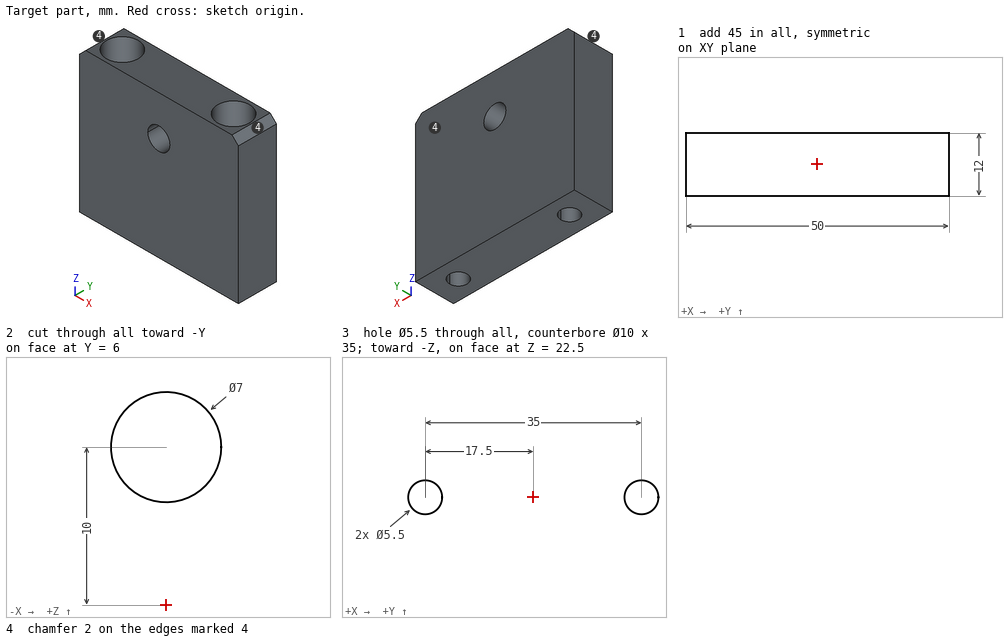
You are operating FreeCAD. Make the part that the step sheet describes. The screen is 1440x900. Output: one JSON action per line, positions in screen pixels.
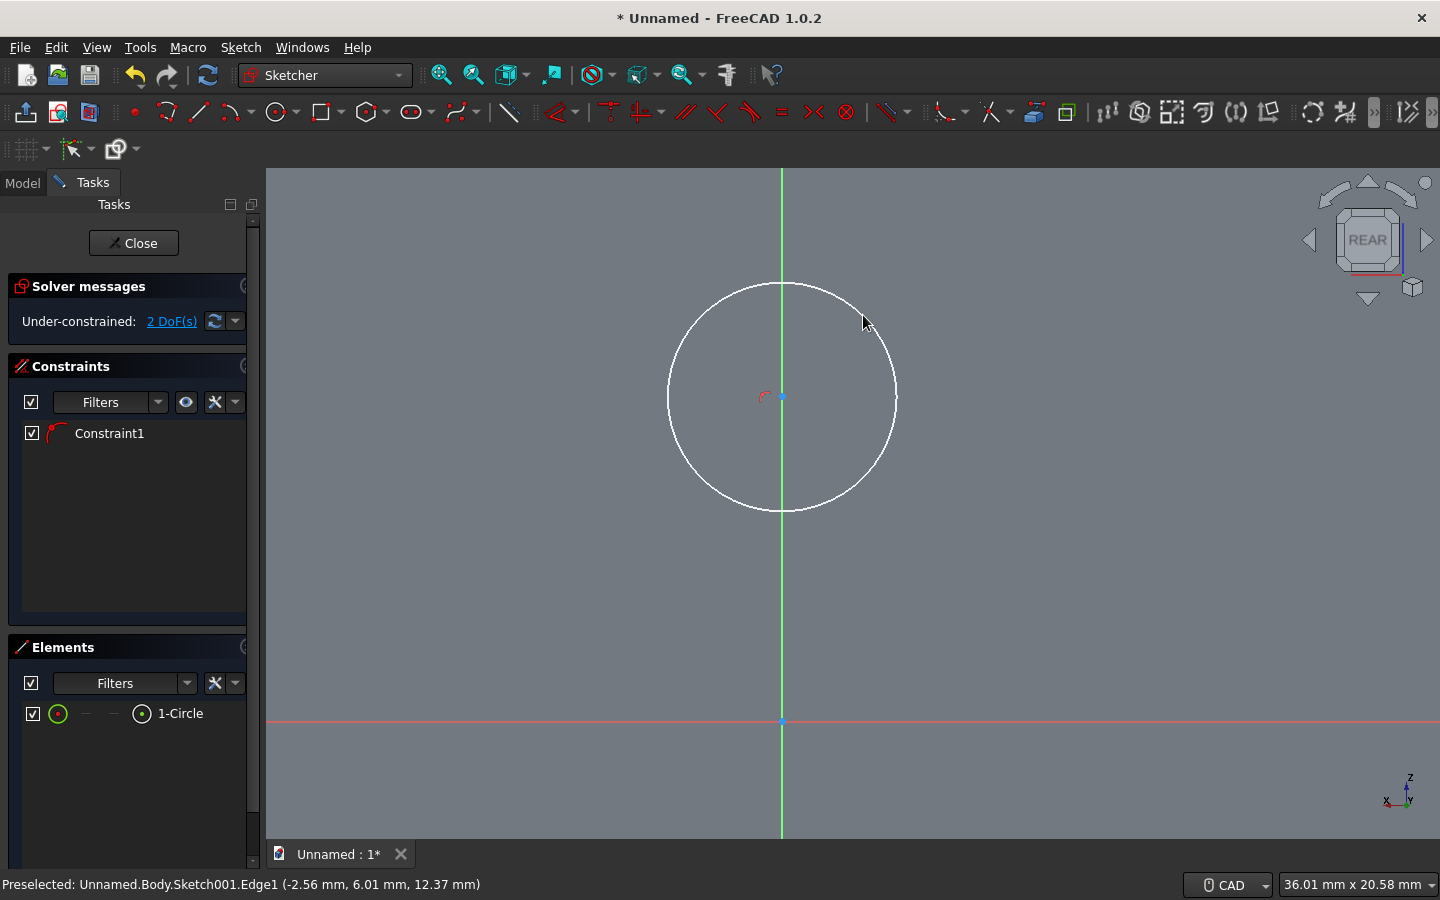
{"action": "left_click", "coordinate": [556, 112]}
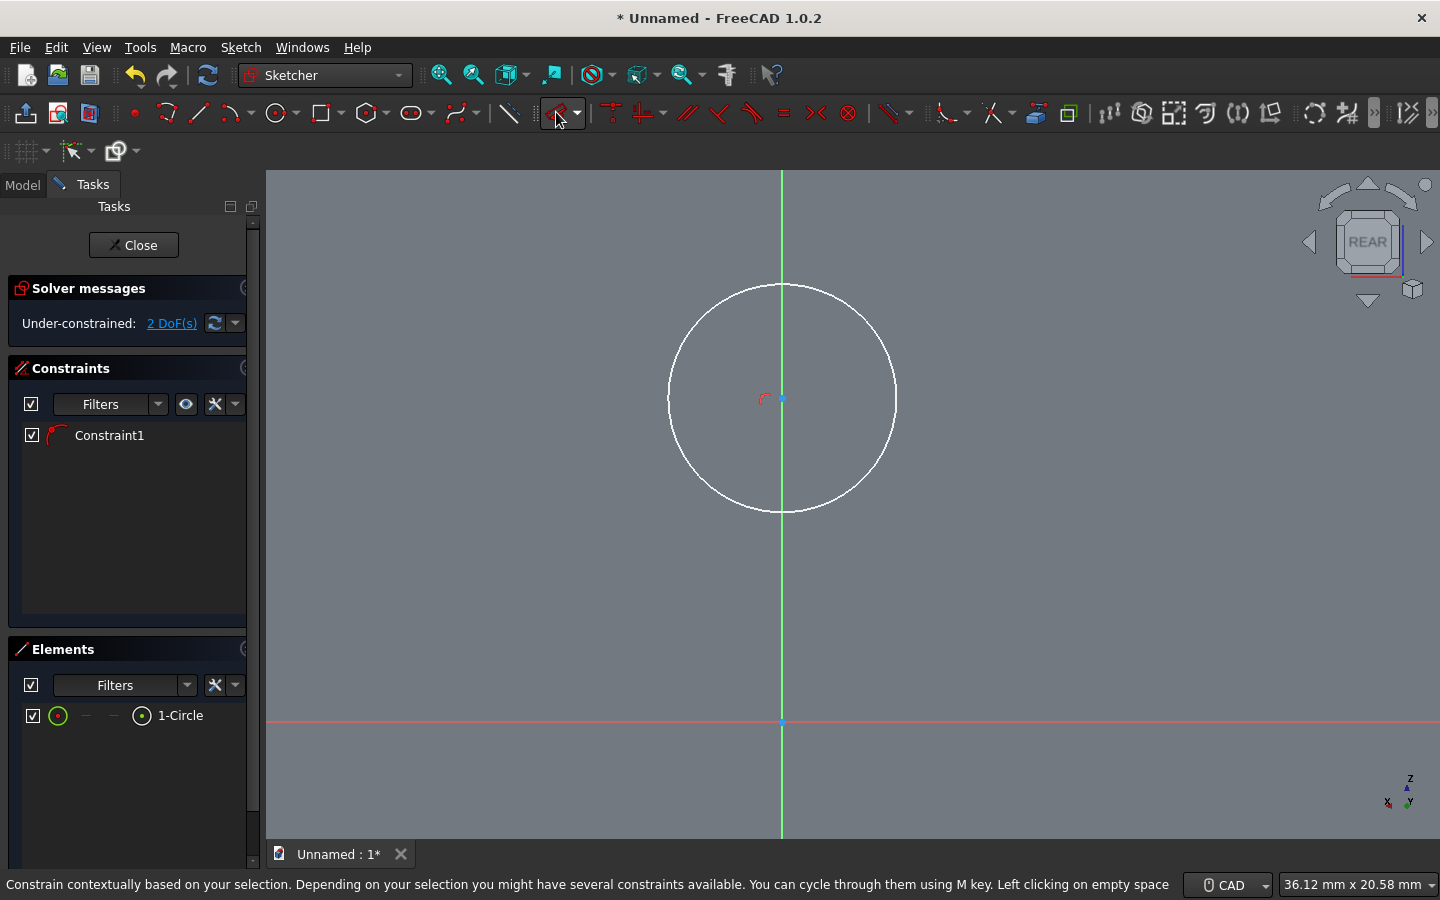
{"action": "left_click", "coordinate": [863, 317]}
{"action": "left_click", "coordinate": [886, 294]}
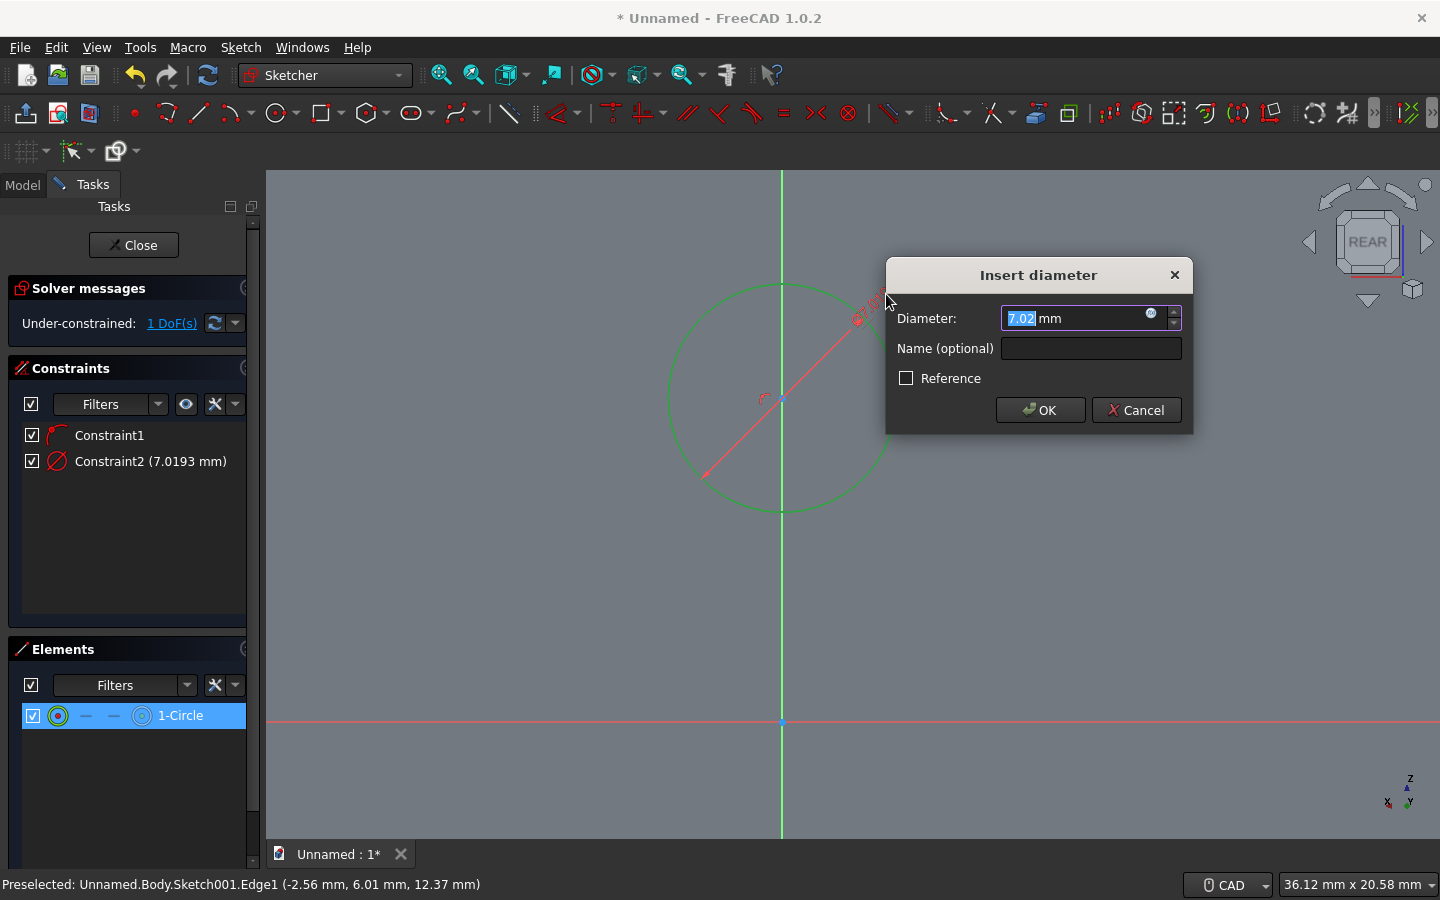
{"action": "type", "text": "7"}
{"action": "key", "text": "Return"}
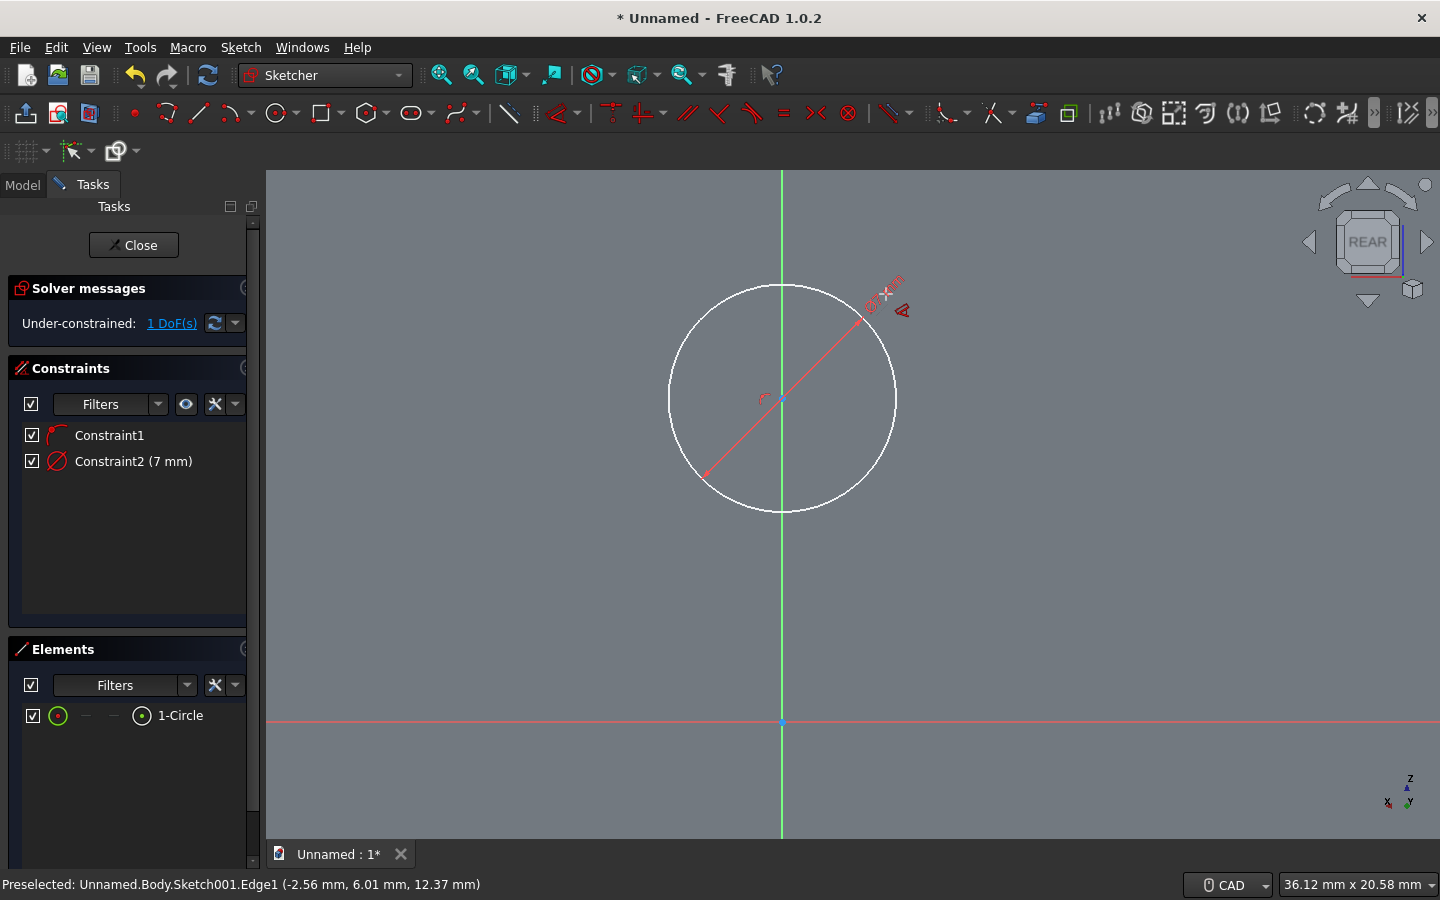
{"action": "left_click", "coordinate": [782, 398]}
{"action": "left_click", "coordinate": [816, 560]}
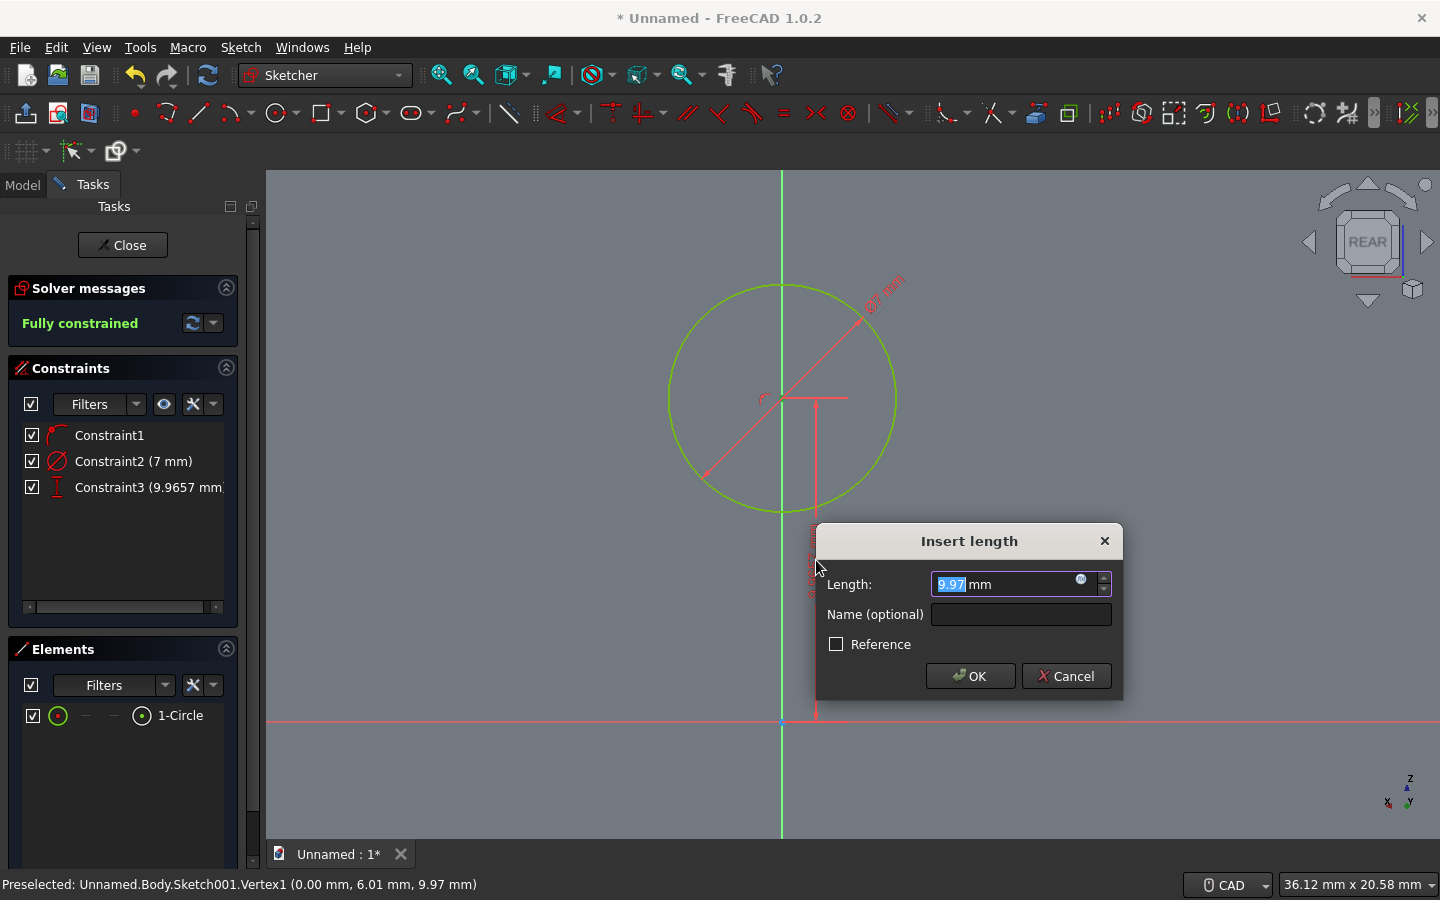
{"action": "type", "text": "10"}
{"action": "key", "text": "Return"}
{"action": "key", "text": "Escape"}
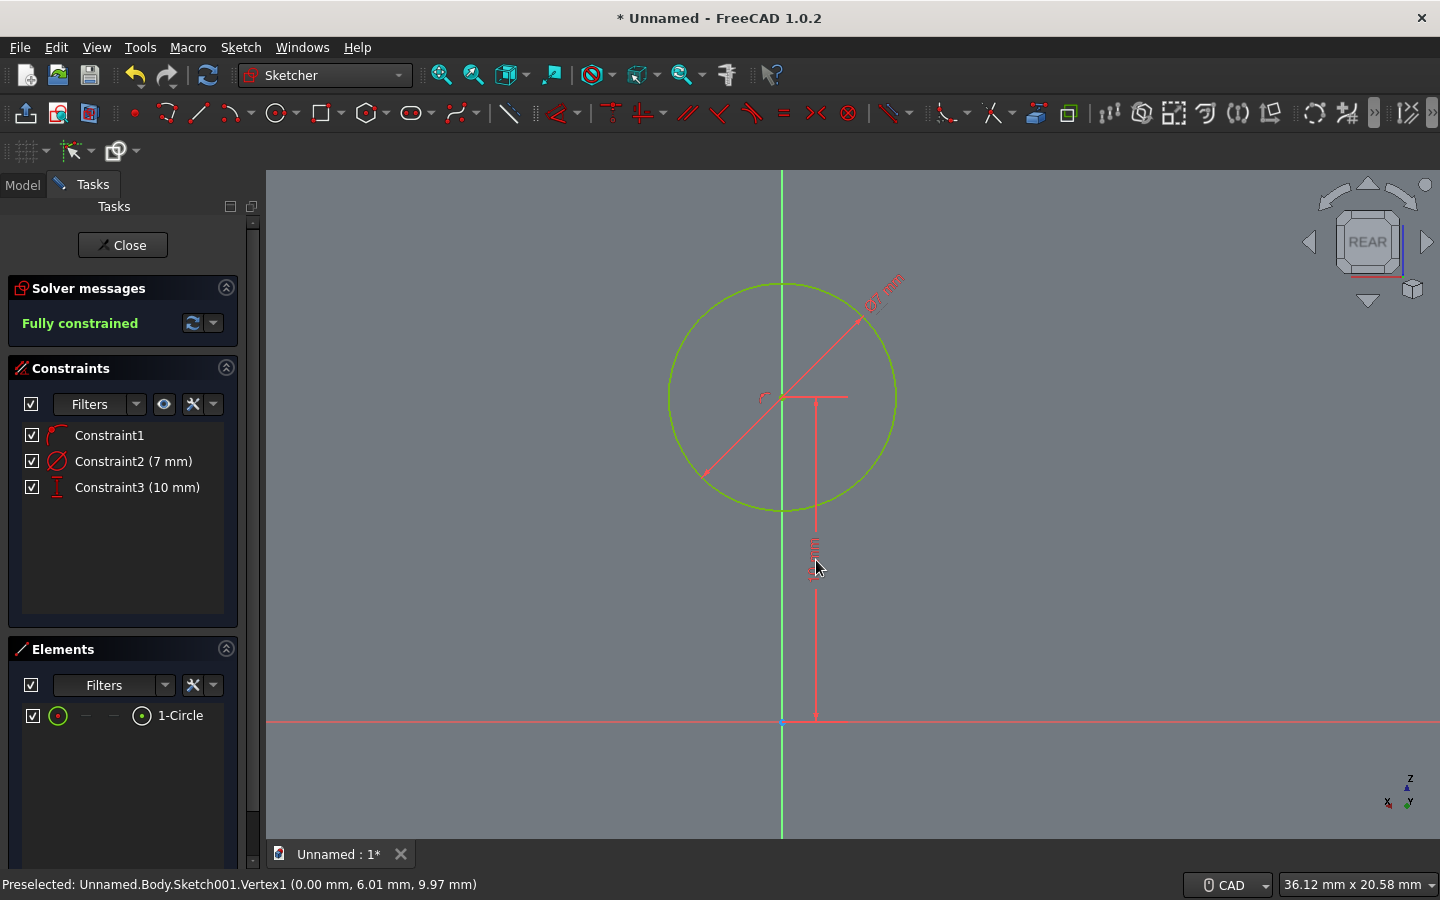
{"action": "left_click", "coordinate": [123, 245]}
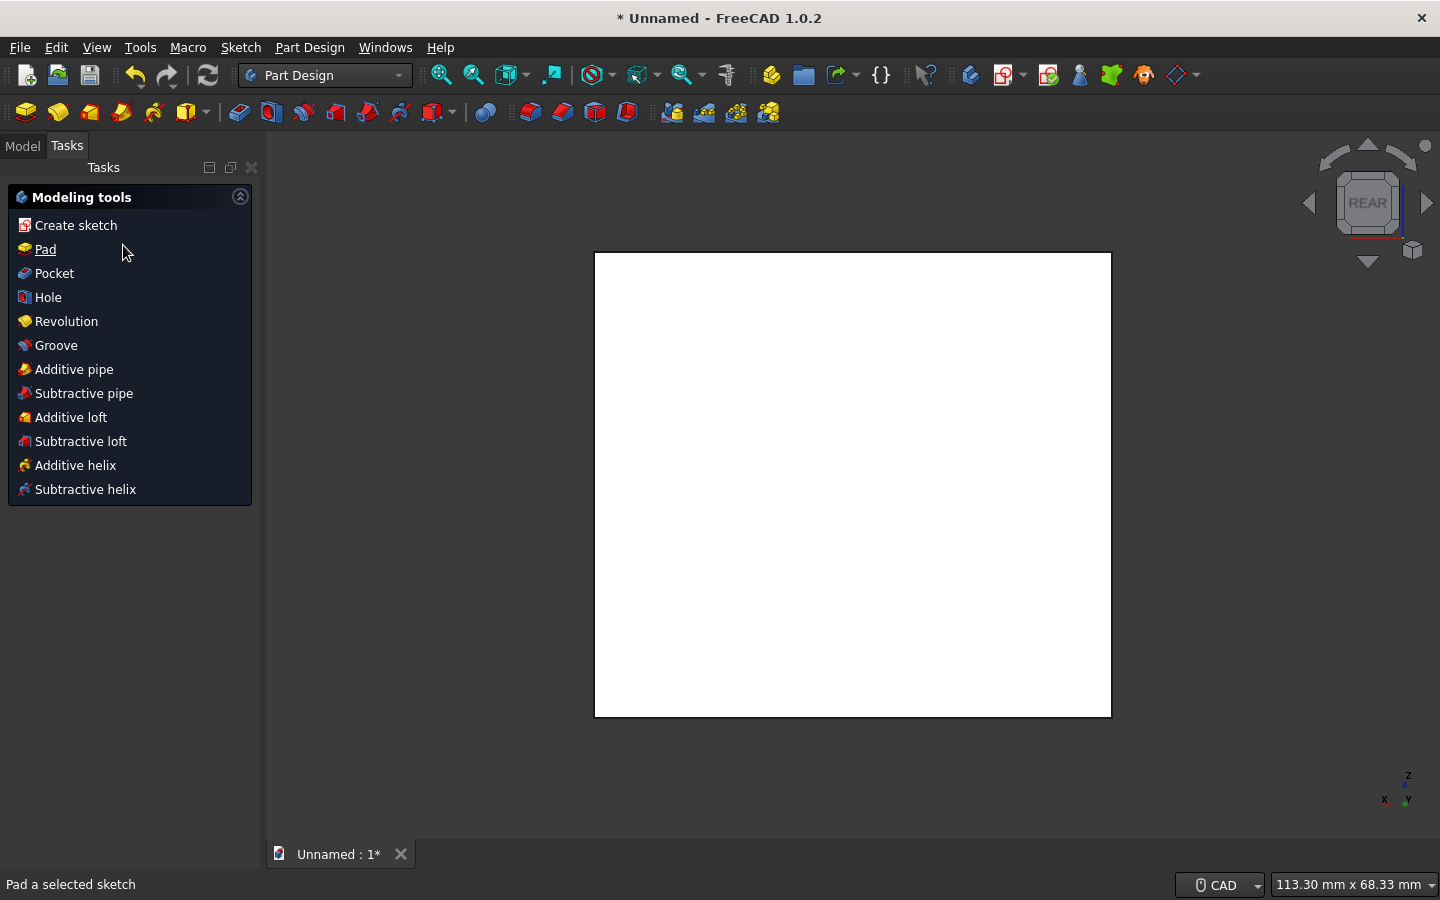
{"action": "left_click", "coordinate": [240, 112]}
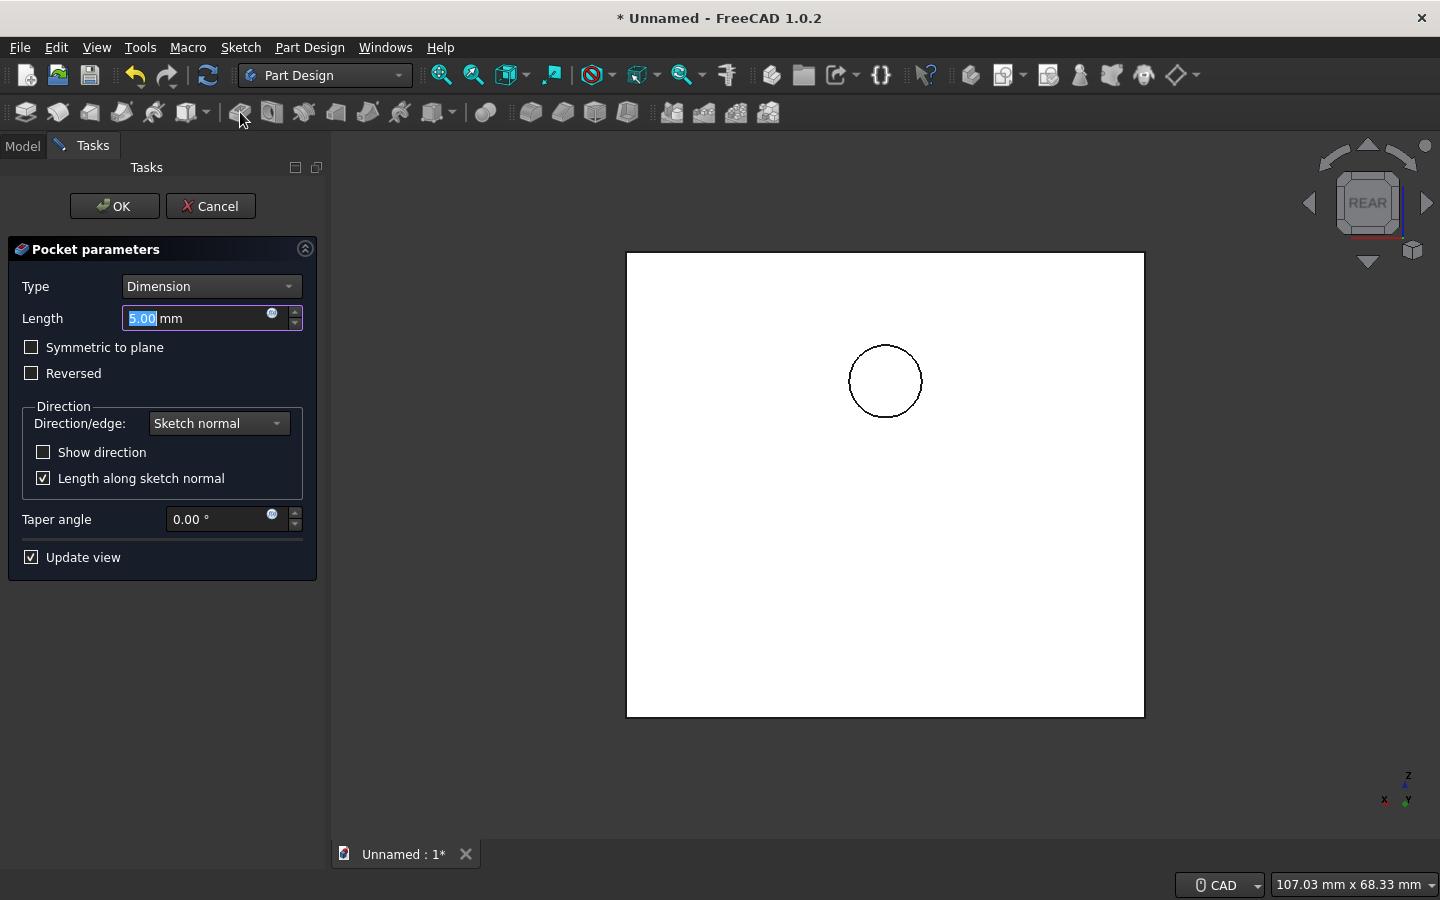
{"action": "left_click", "coordinate": [212, 286]}